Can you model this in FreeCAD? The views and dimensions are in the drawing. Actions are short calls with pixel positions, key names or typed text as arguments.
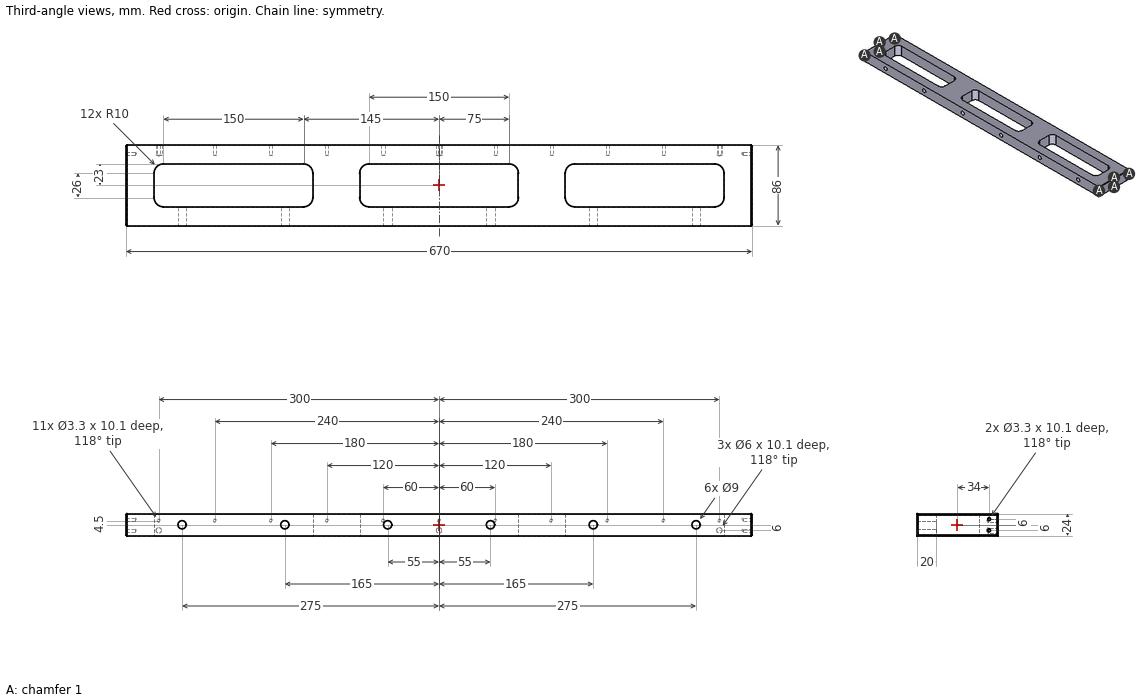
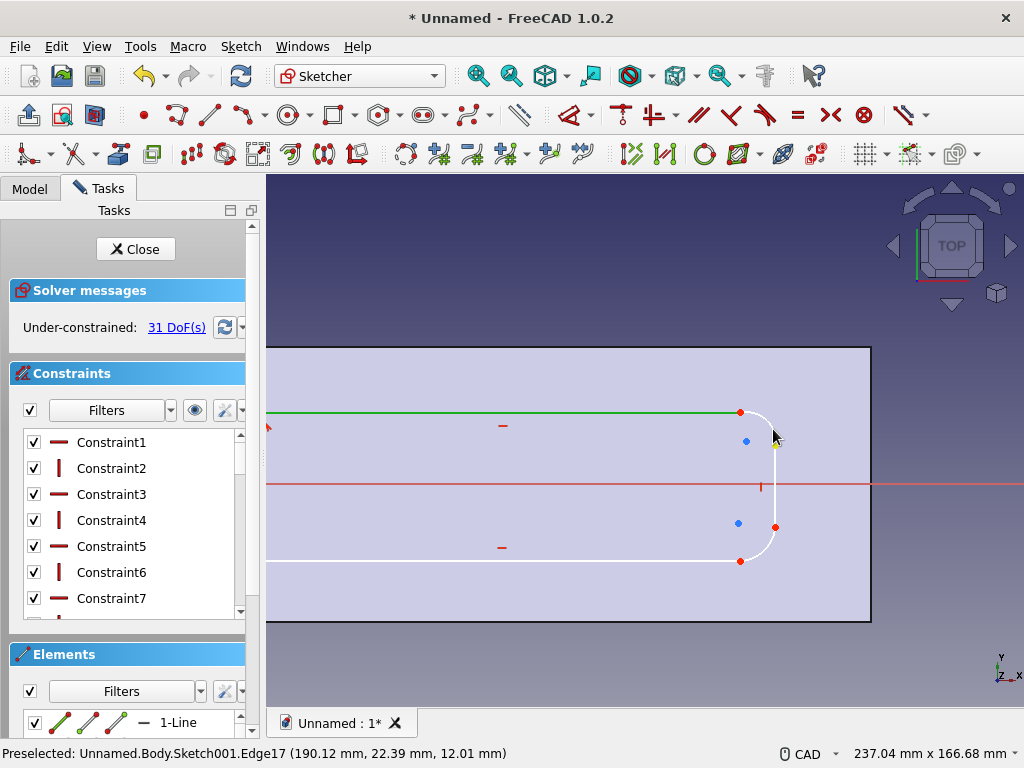
click(773, 429)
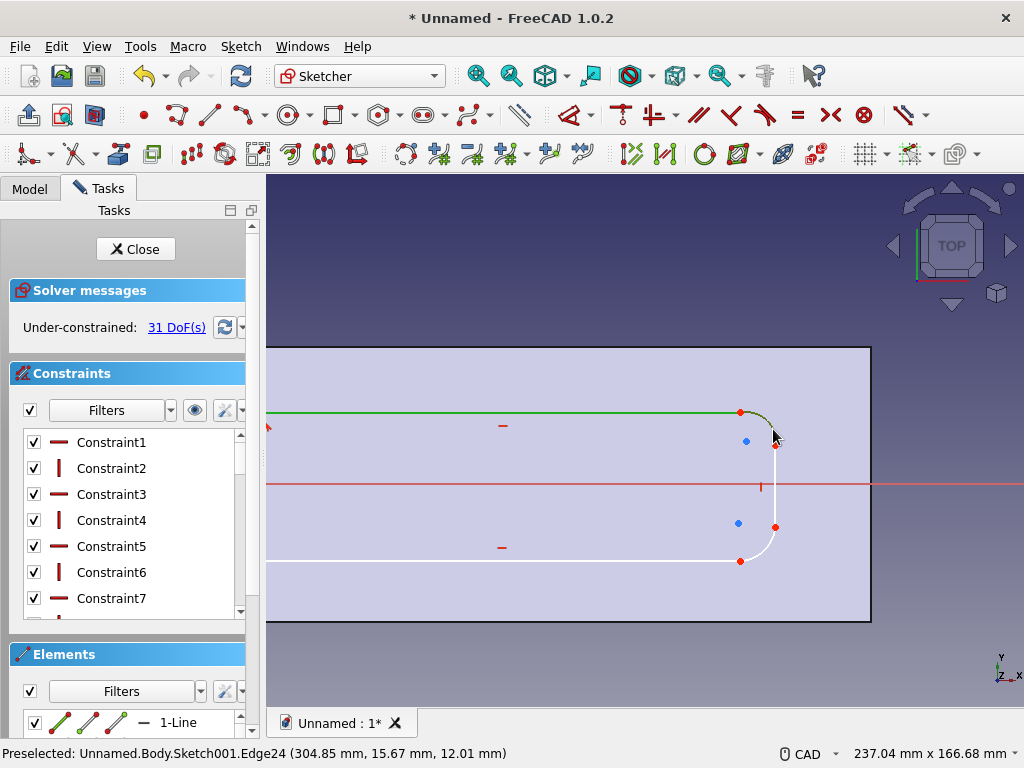
key(t)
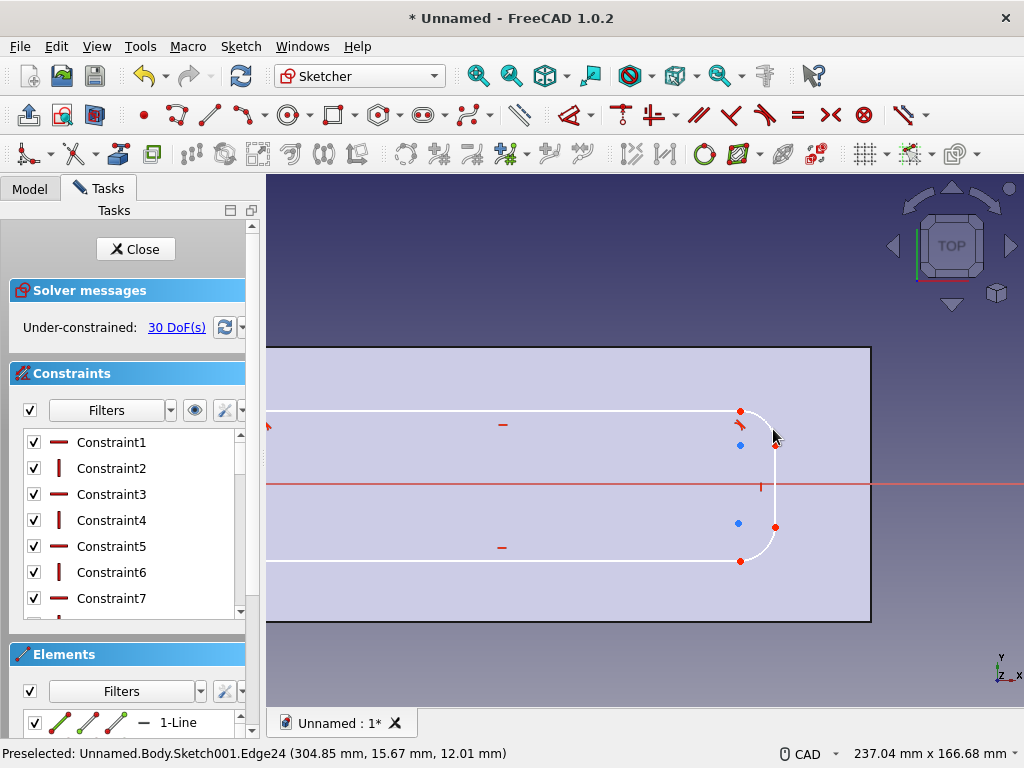
scroll(773, 429, down, 8)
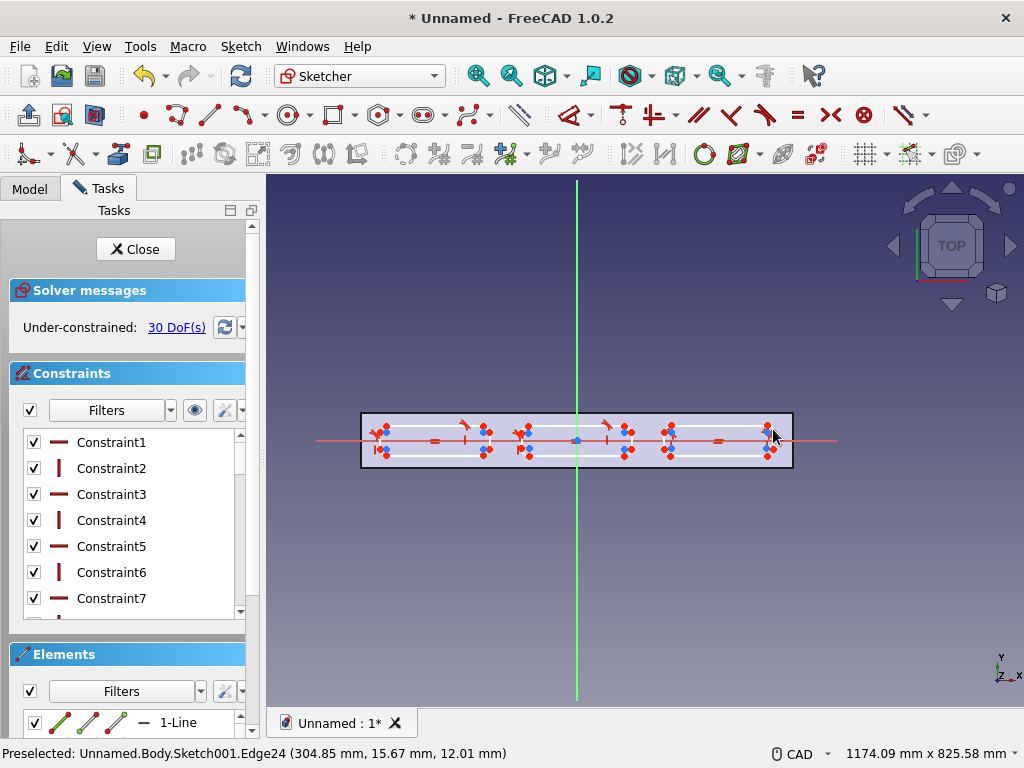
scroll(664, 438, up, 8)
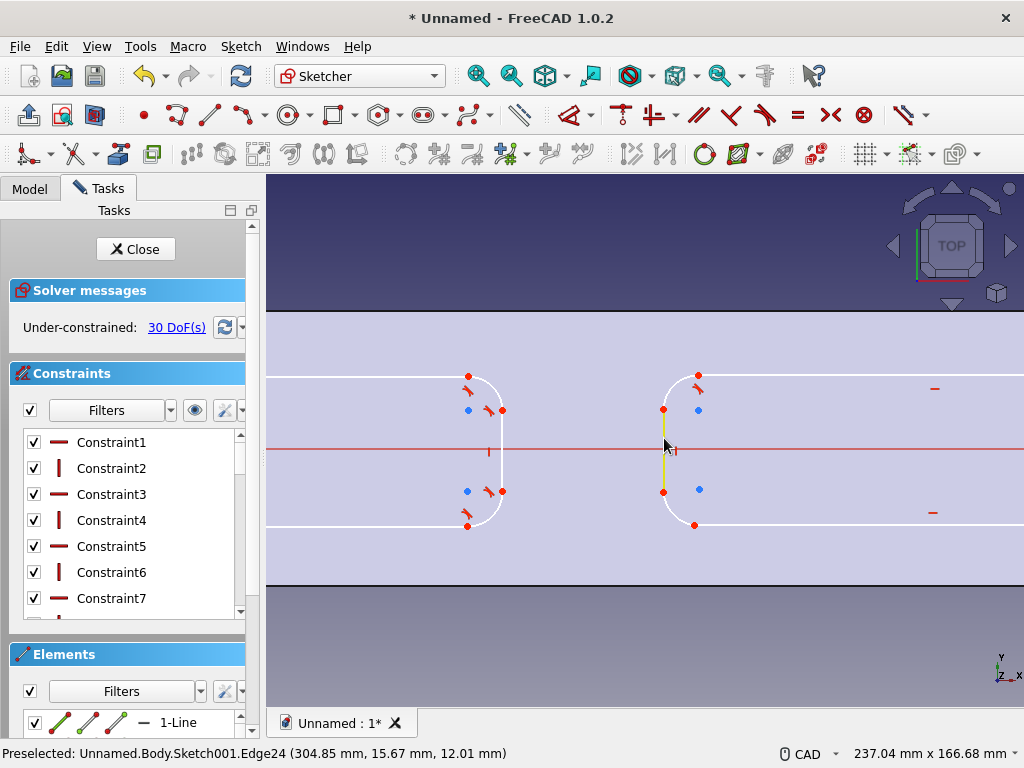
click(664, 434)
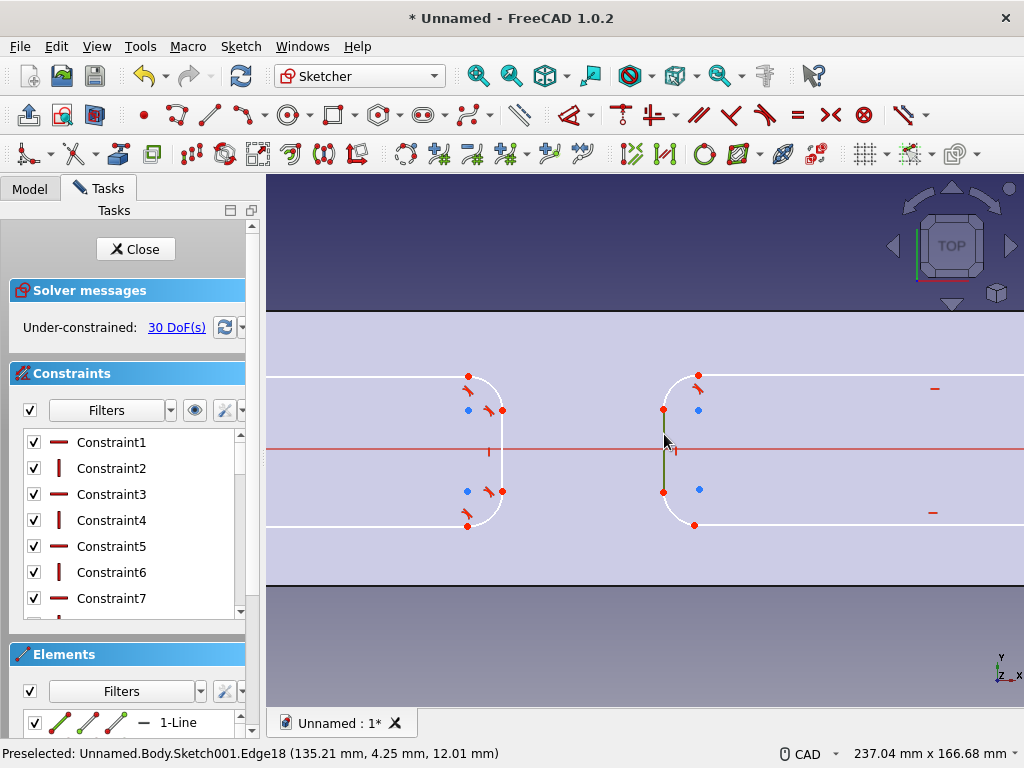
click(683, 379)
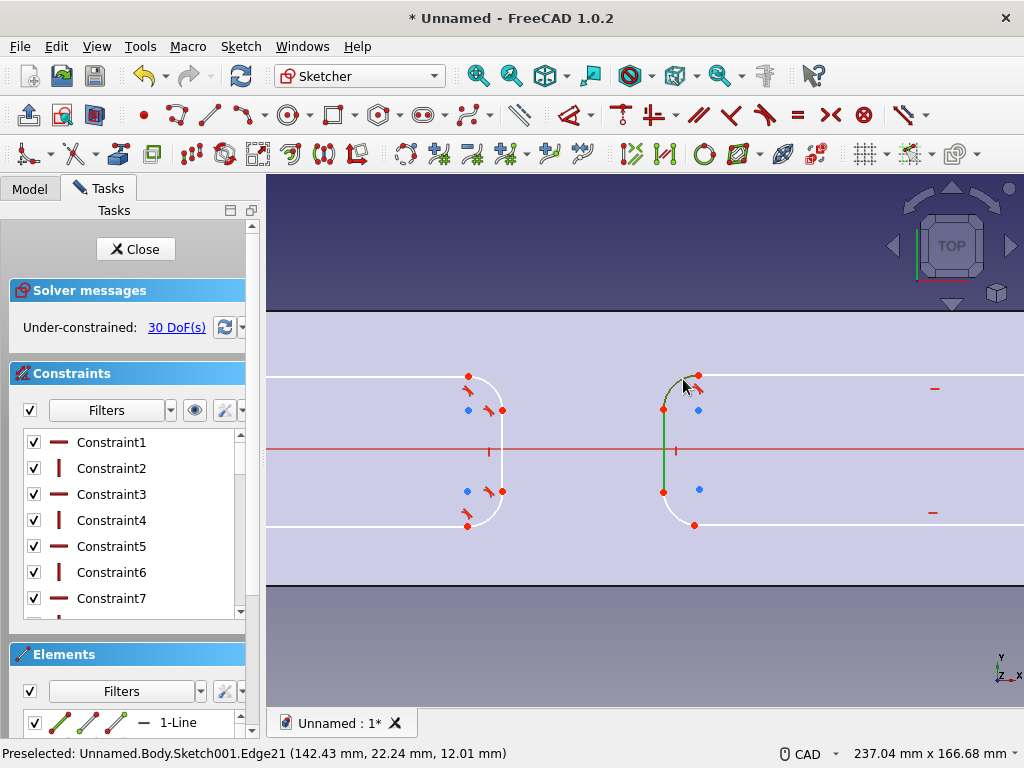
key(t)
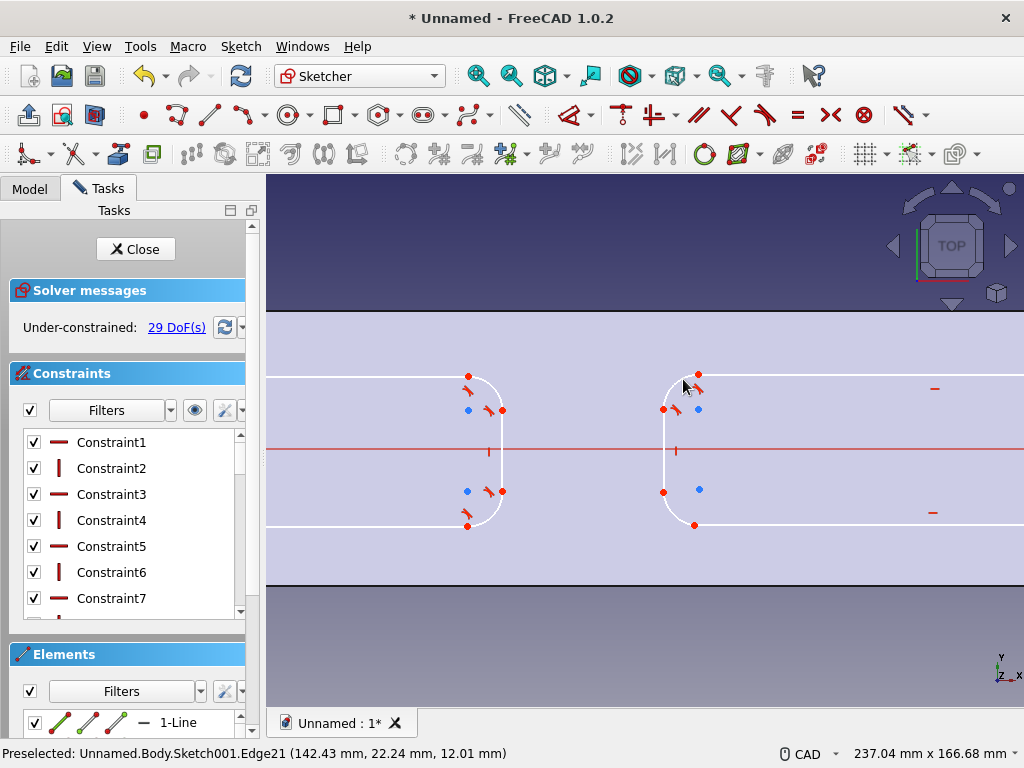
click(664, 434)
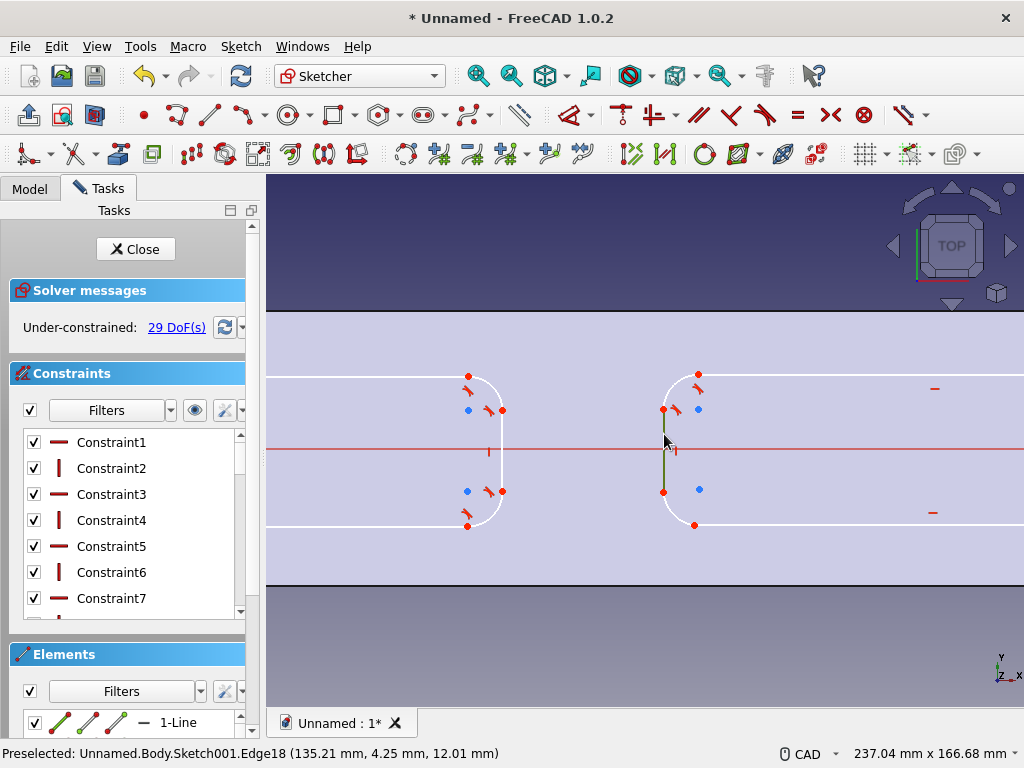
click(668, 506)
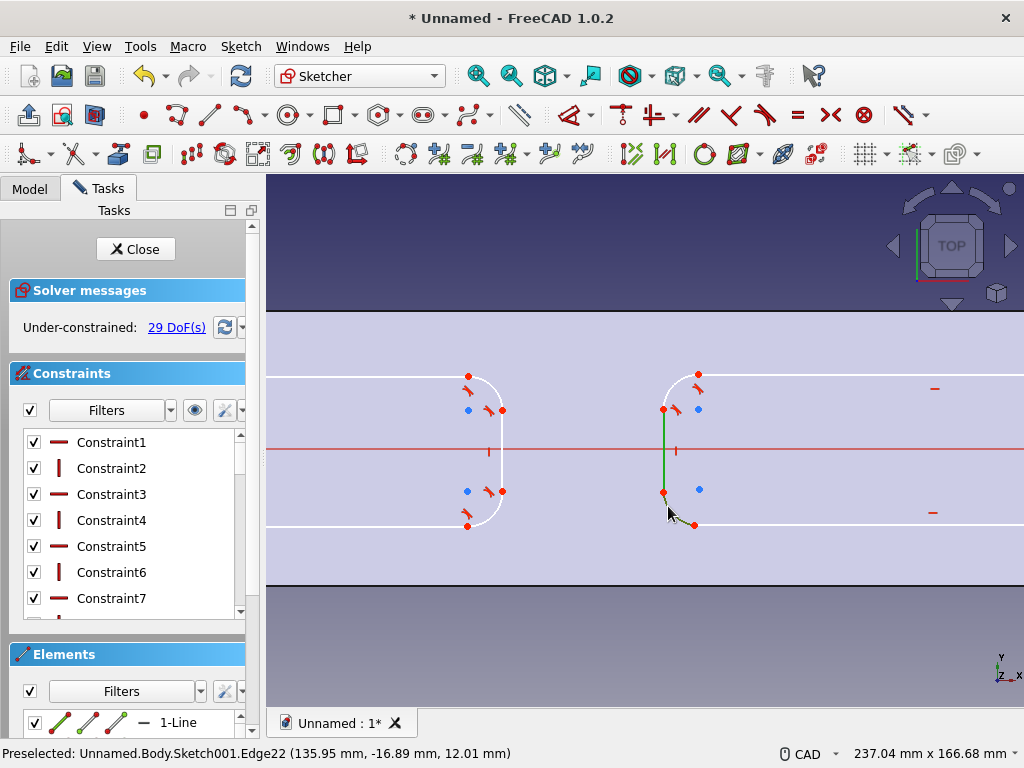
key(t)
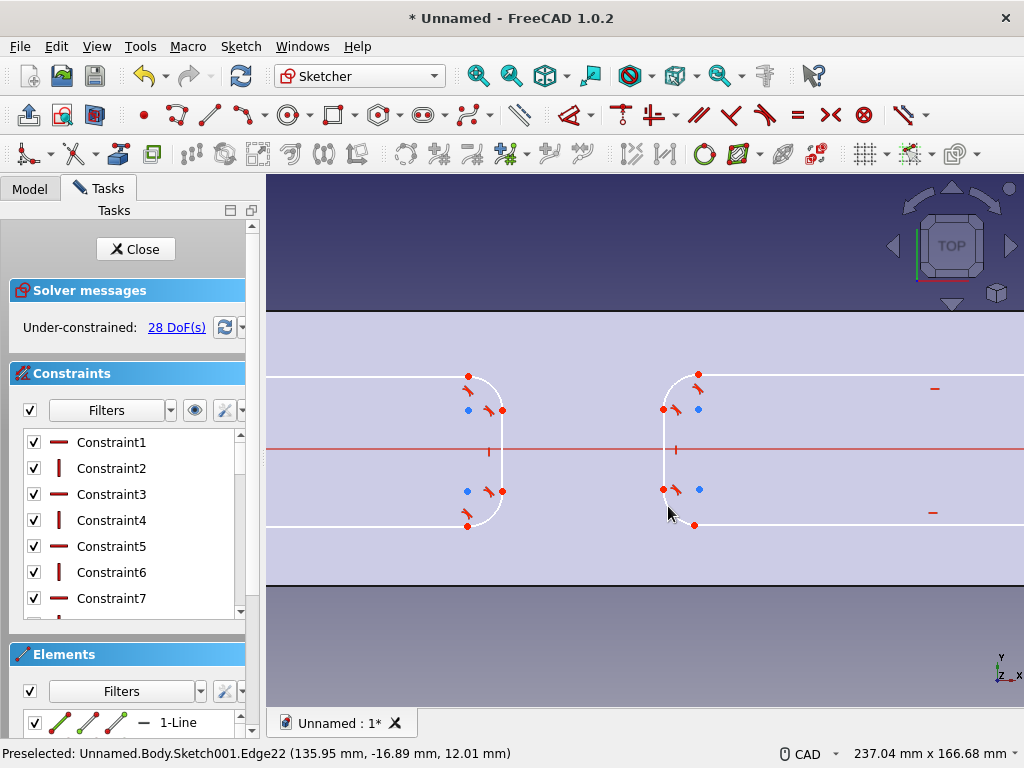
scroll(664, 438, down, 8)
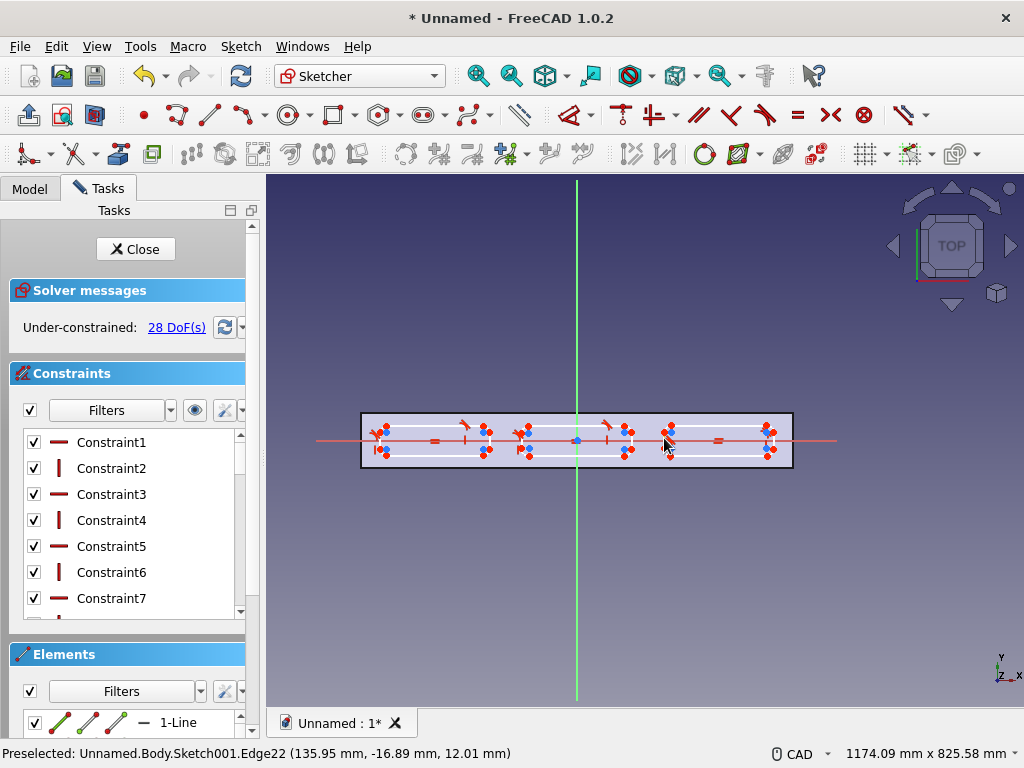
click(700, 456)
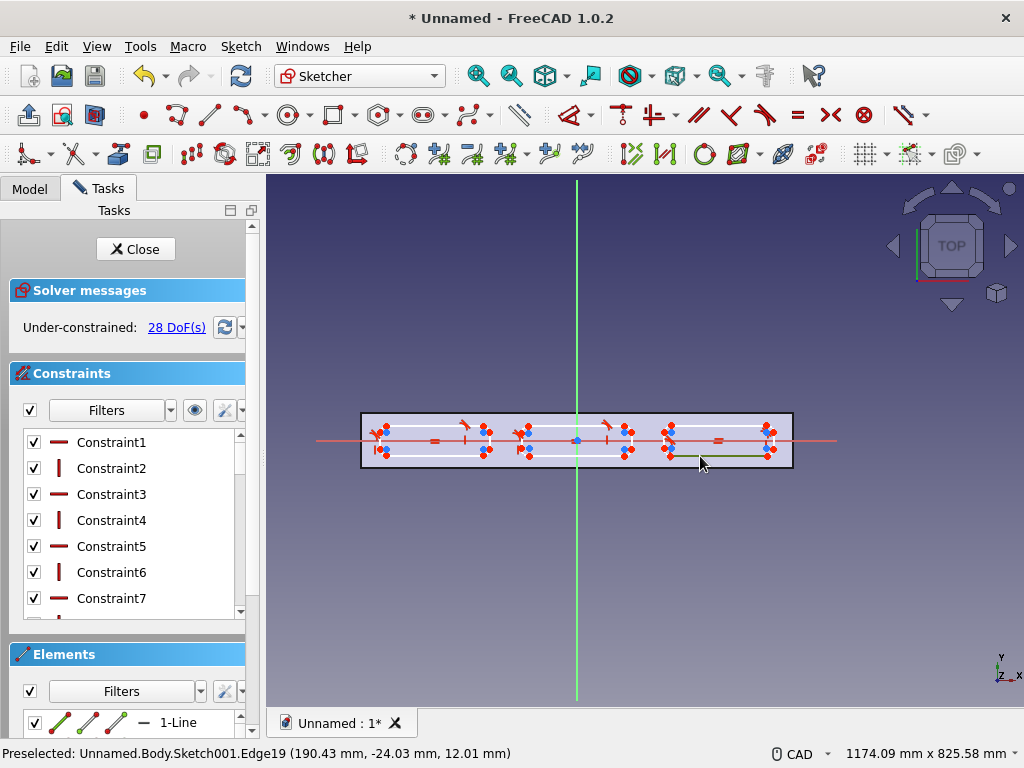
scroll(666, 454, up, 5)